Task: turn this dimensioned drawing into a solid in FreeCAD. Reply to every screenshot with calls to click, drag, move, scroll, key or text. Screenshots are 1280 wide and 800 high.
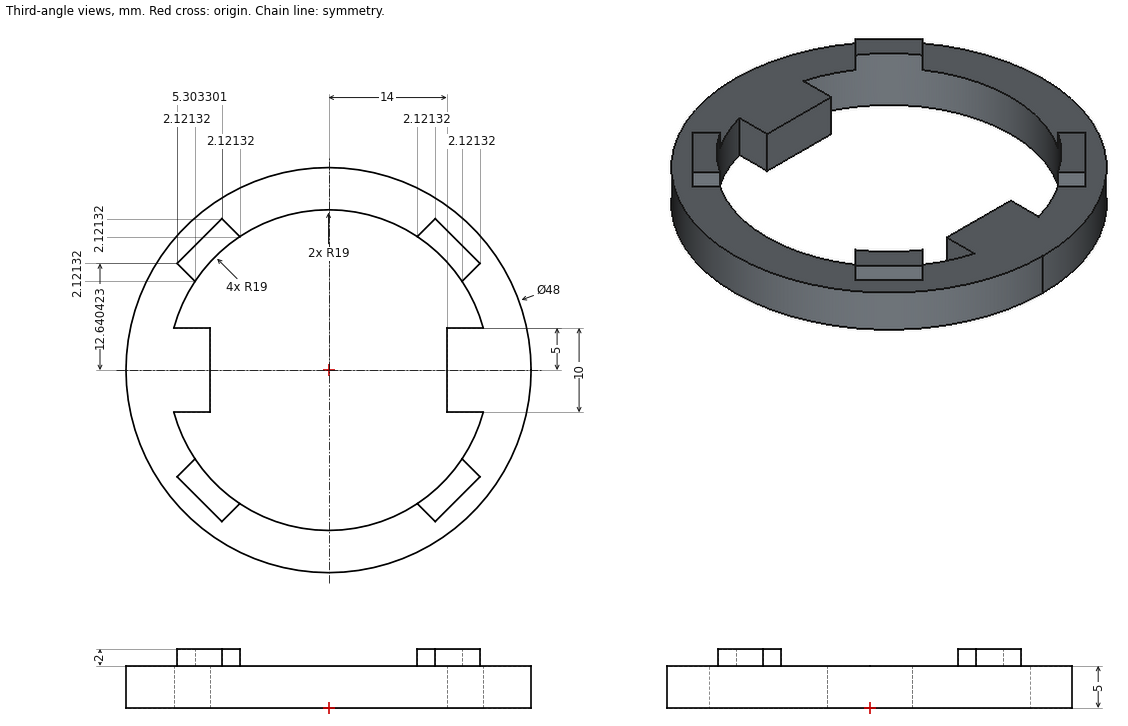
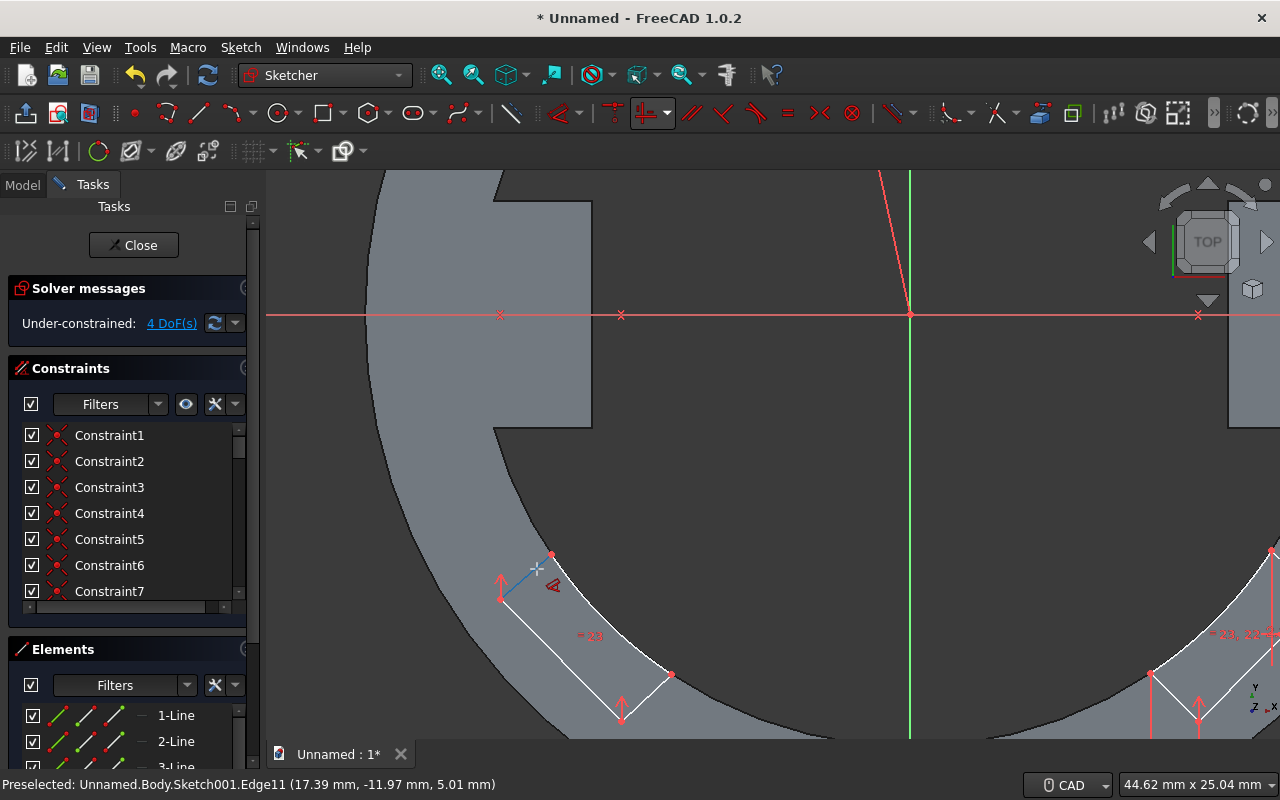
click(536, 568)
click(514, 633)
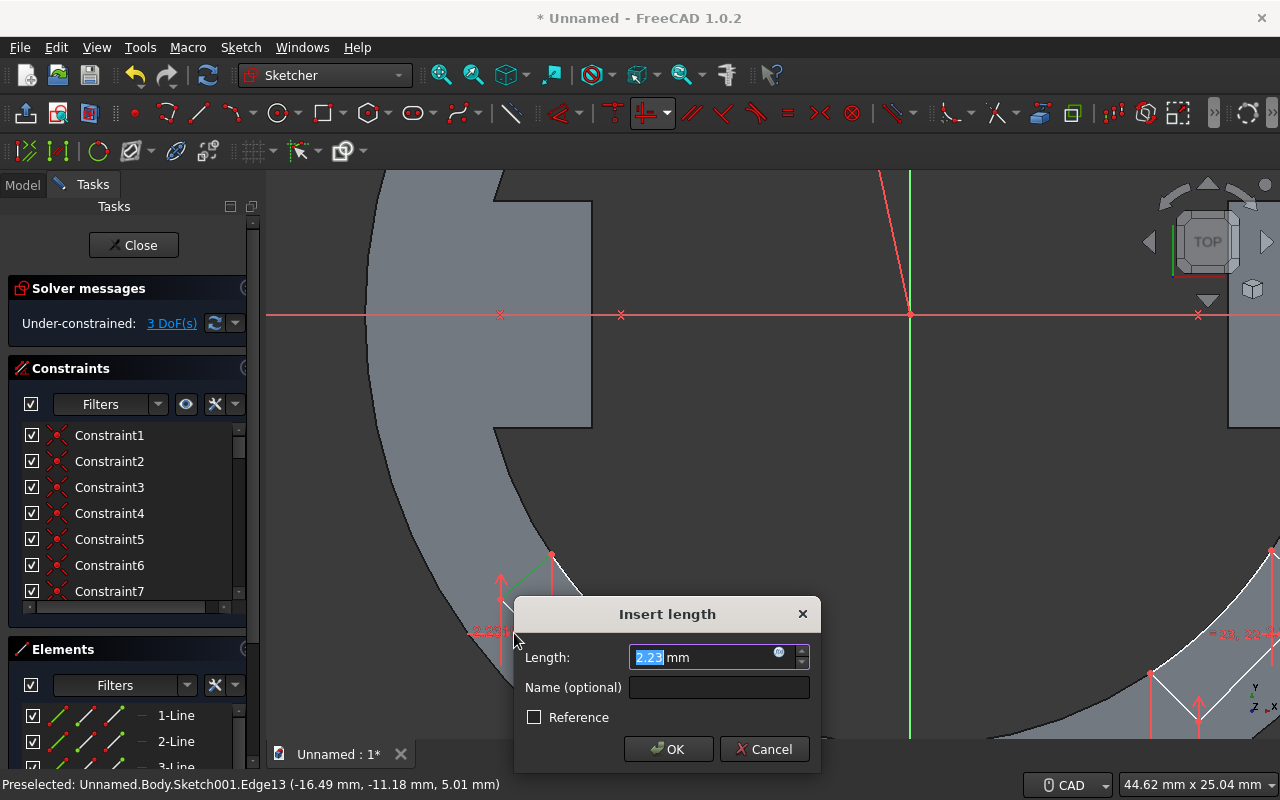
text(2.12132)
key(Return)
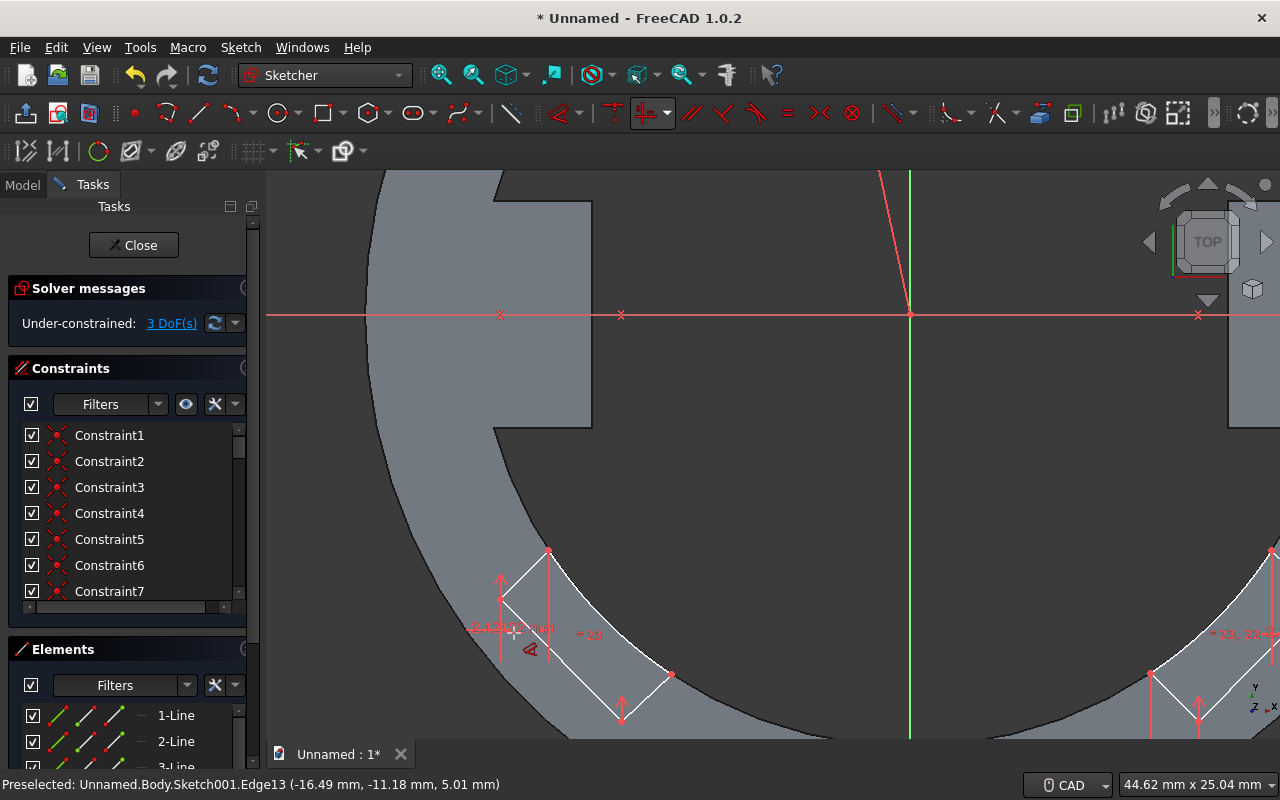
click(637, 707)
click(658, 641)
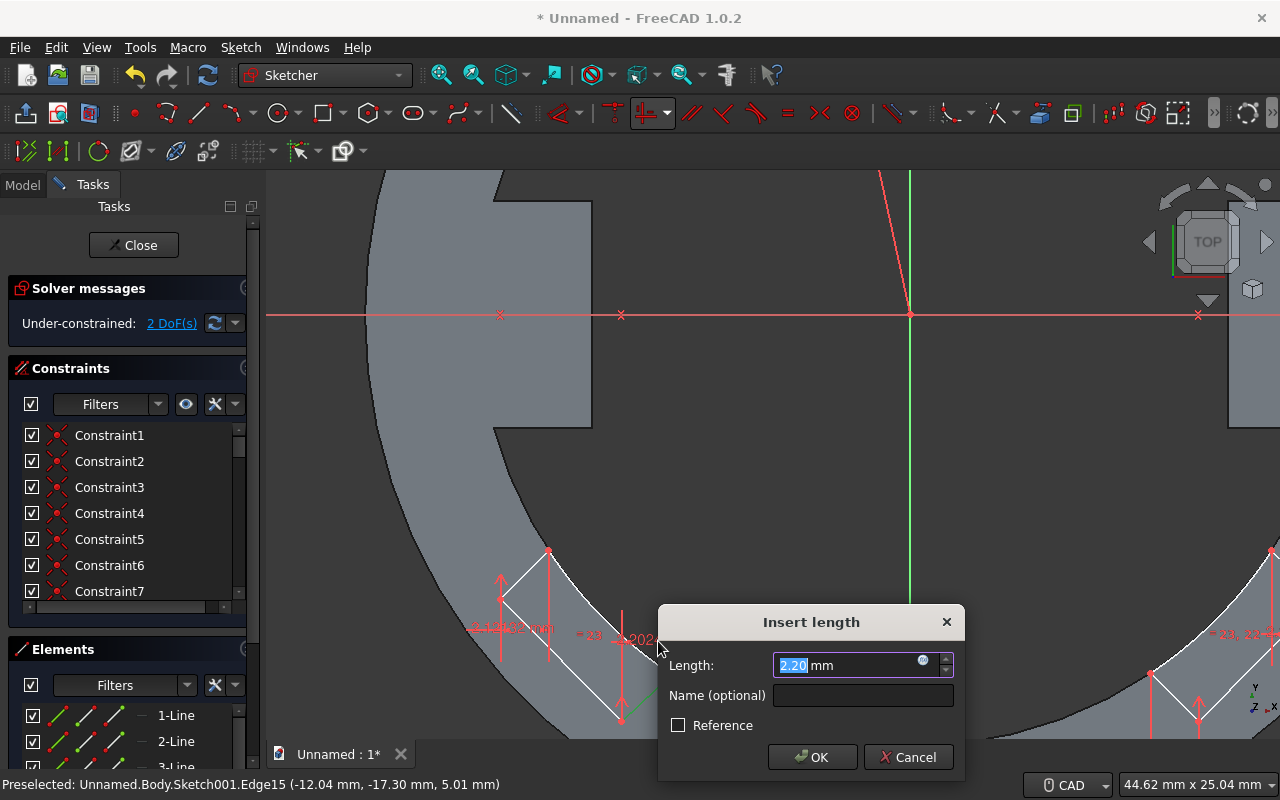
text(2.12132)
key(Return)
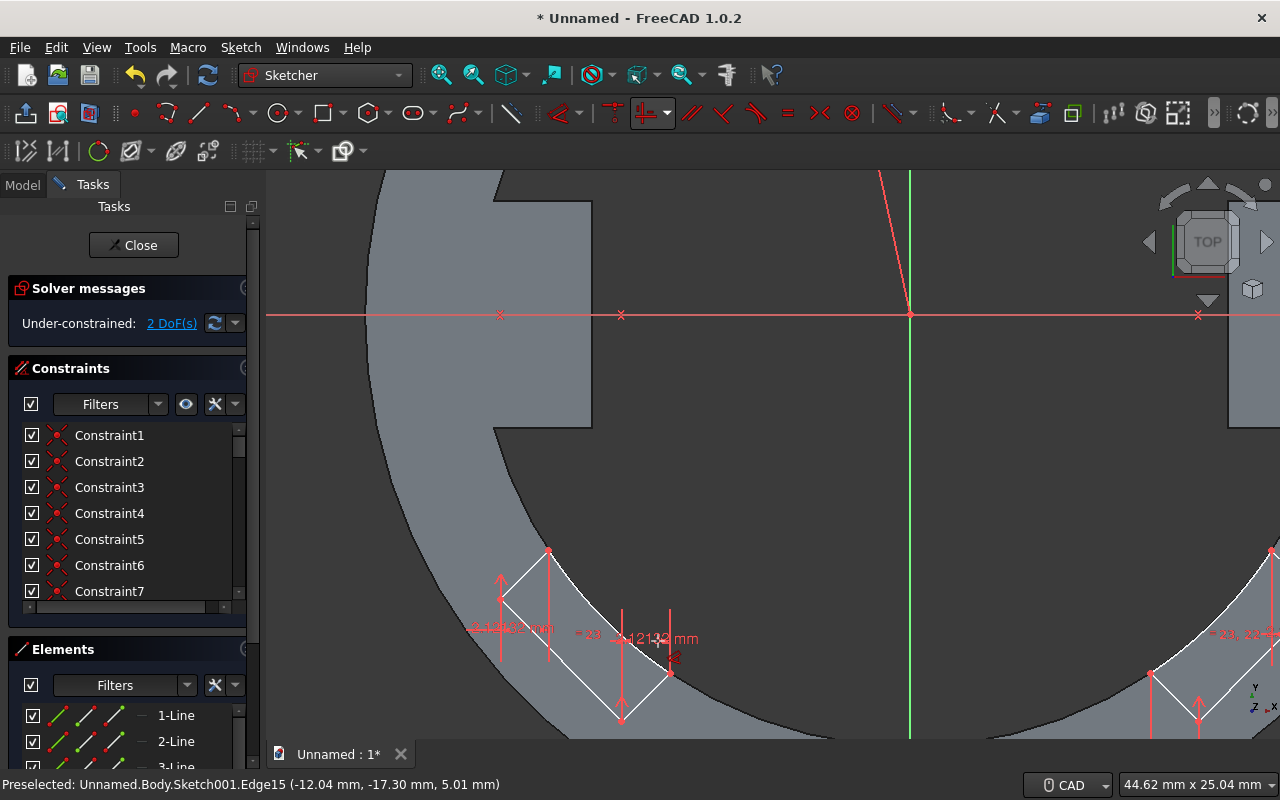
scroll(537, 569, down, 4)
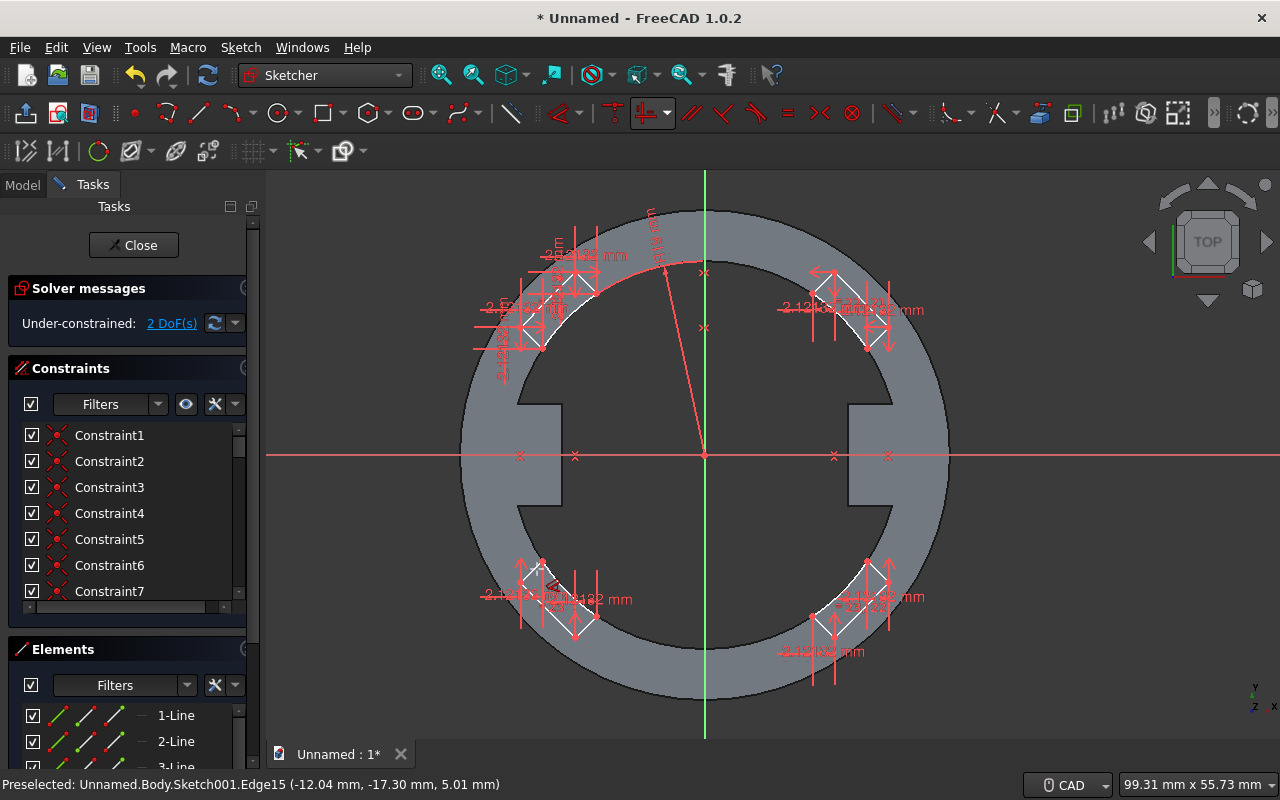
click(559, 289)
click(548, 361)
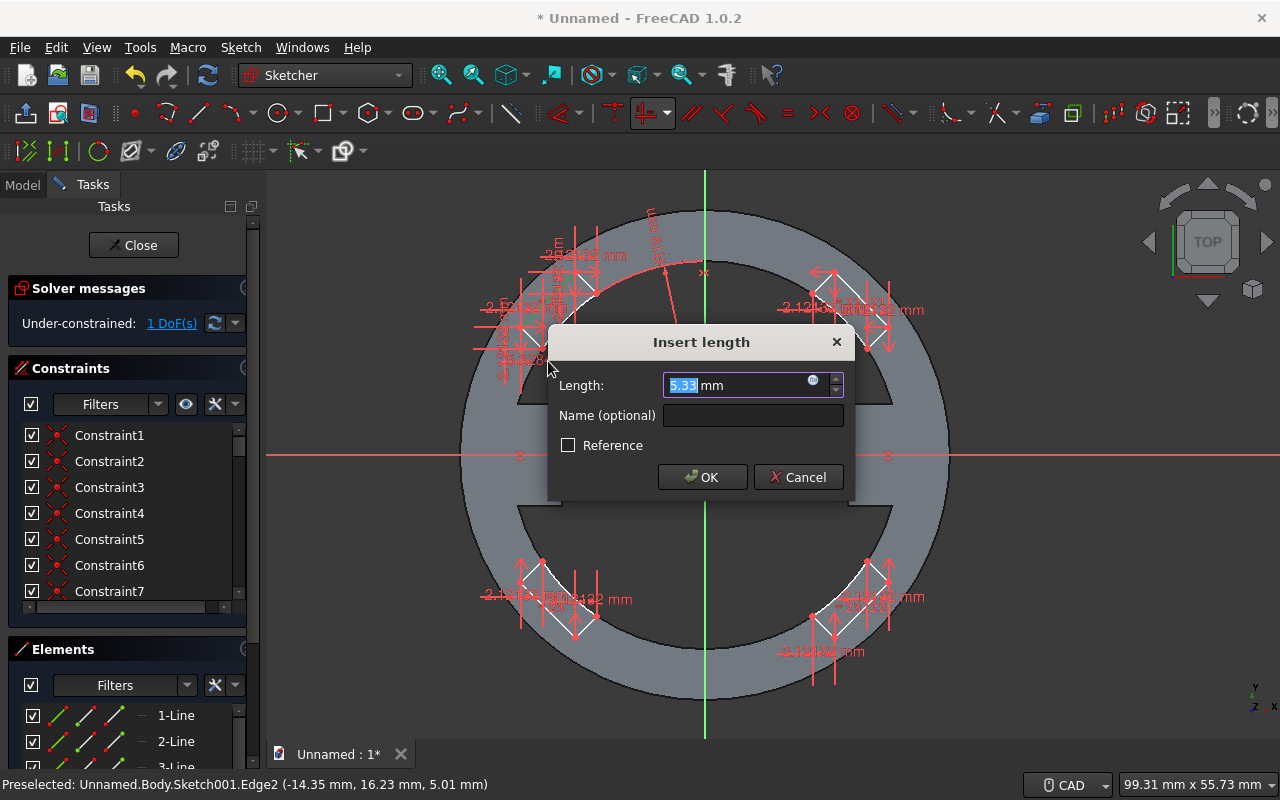
text(5.303301)
key(Return)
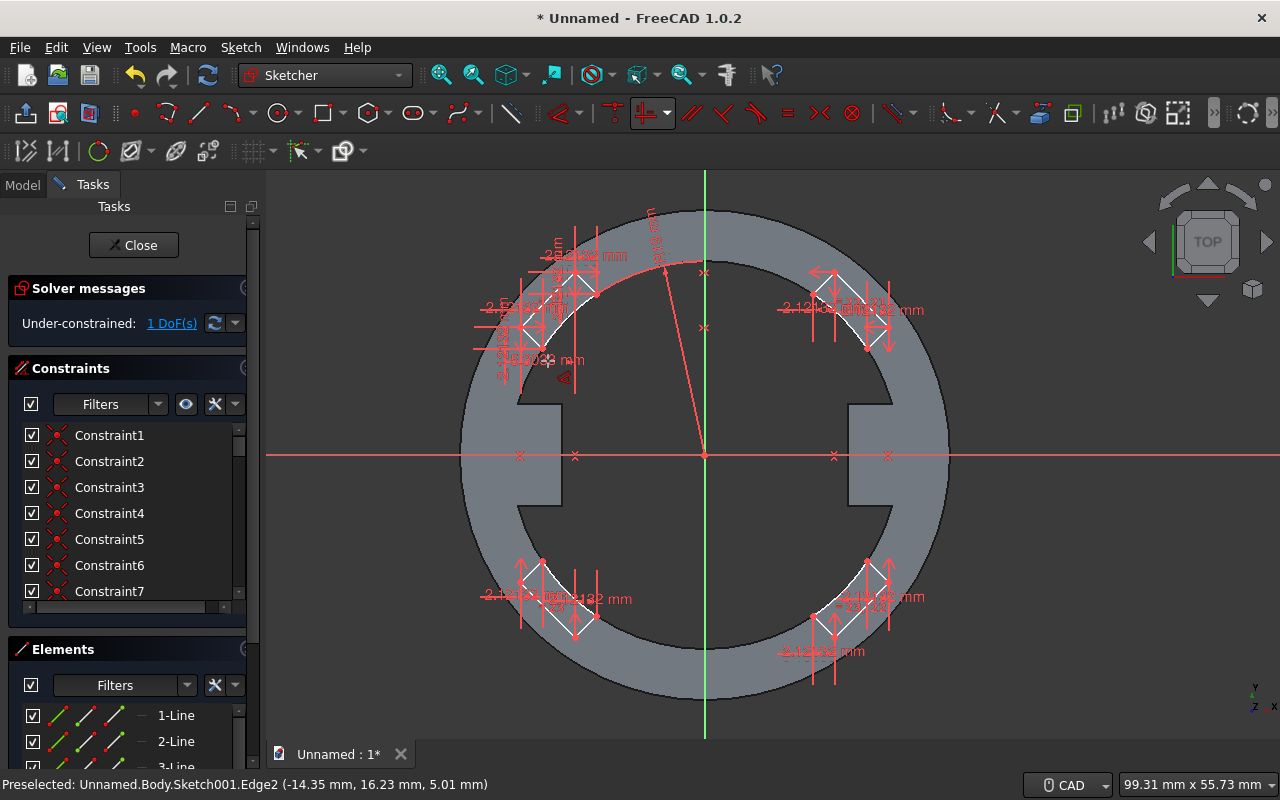
click(521, 327)
click(487, 391)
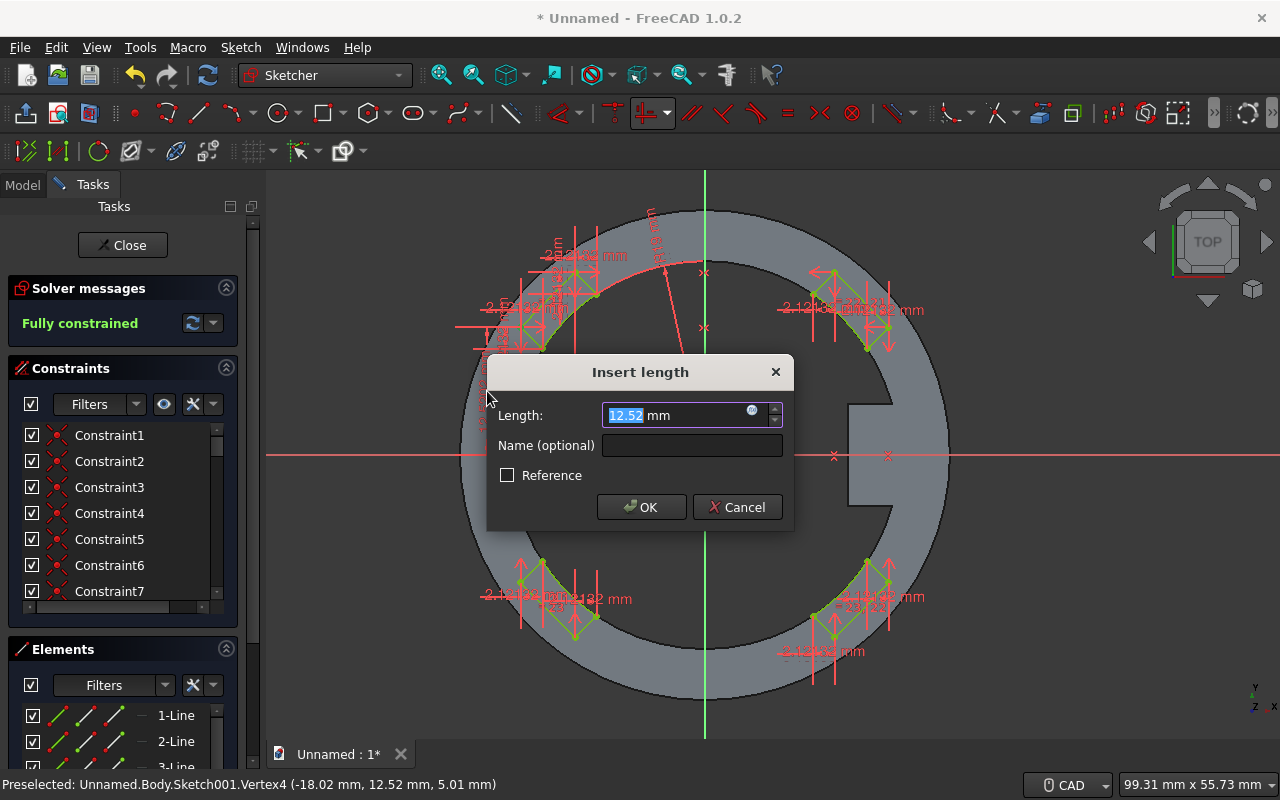
text(12.640423)
key(Return)
key(Escape)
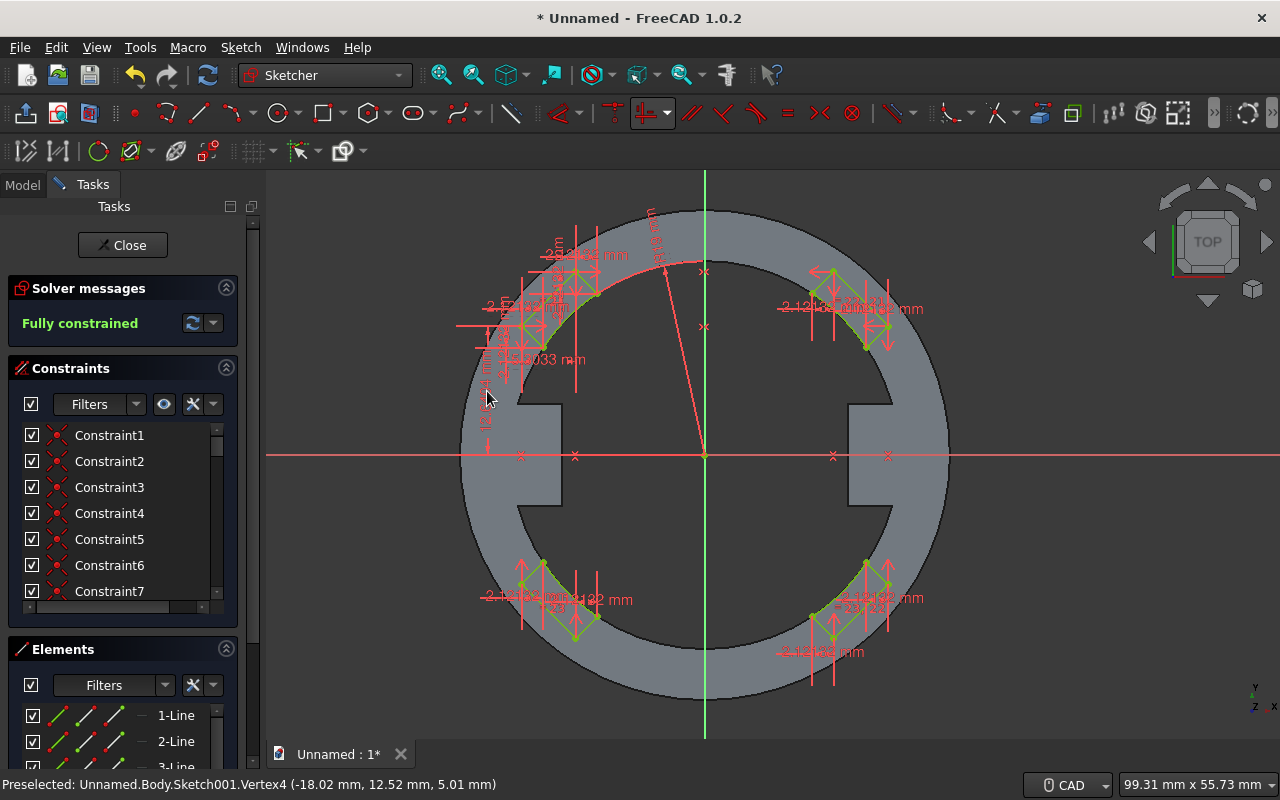
click(123, 245)